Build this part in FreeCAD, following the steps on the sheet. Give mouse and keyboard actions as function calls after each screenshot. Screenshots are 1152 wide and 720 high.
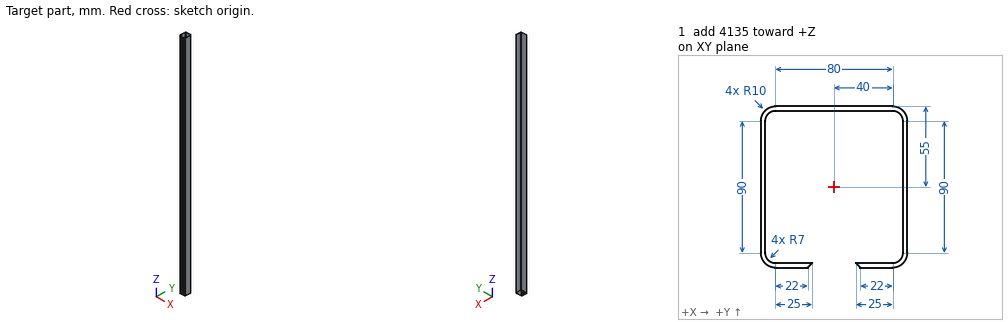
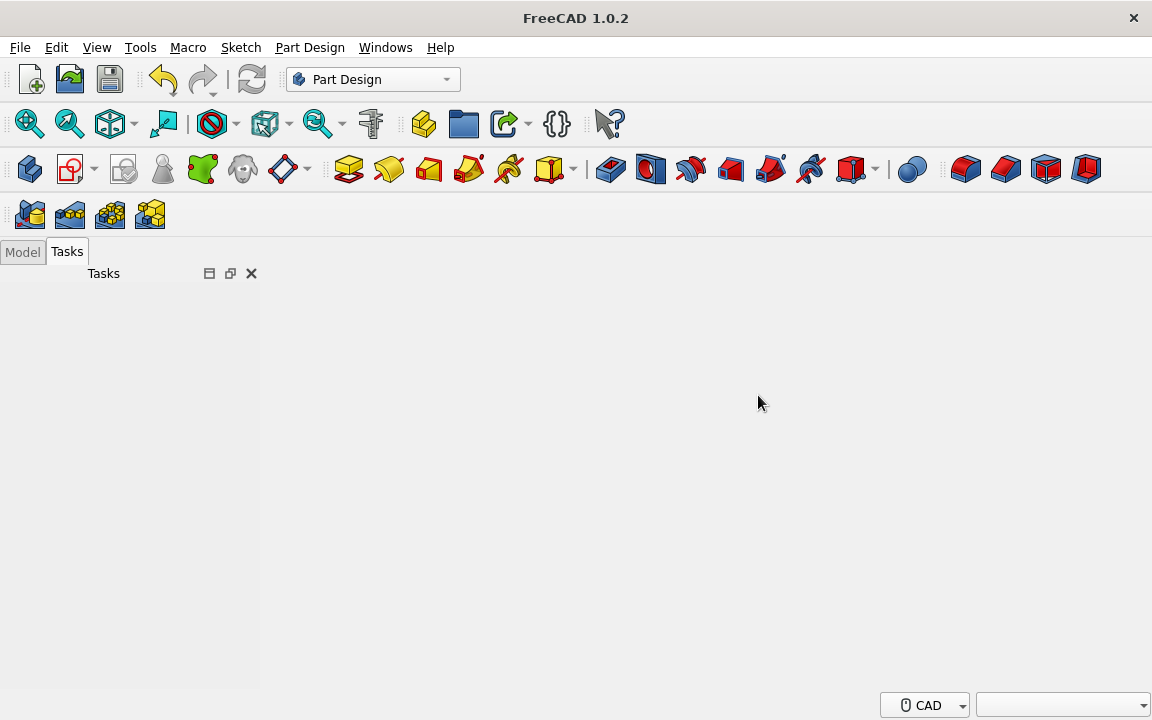
click(30, 80)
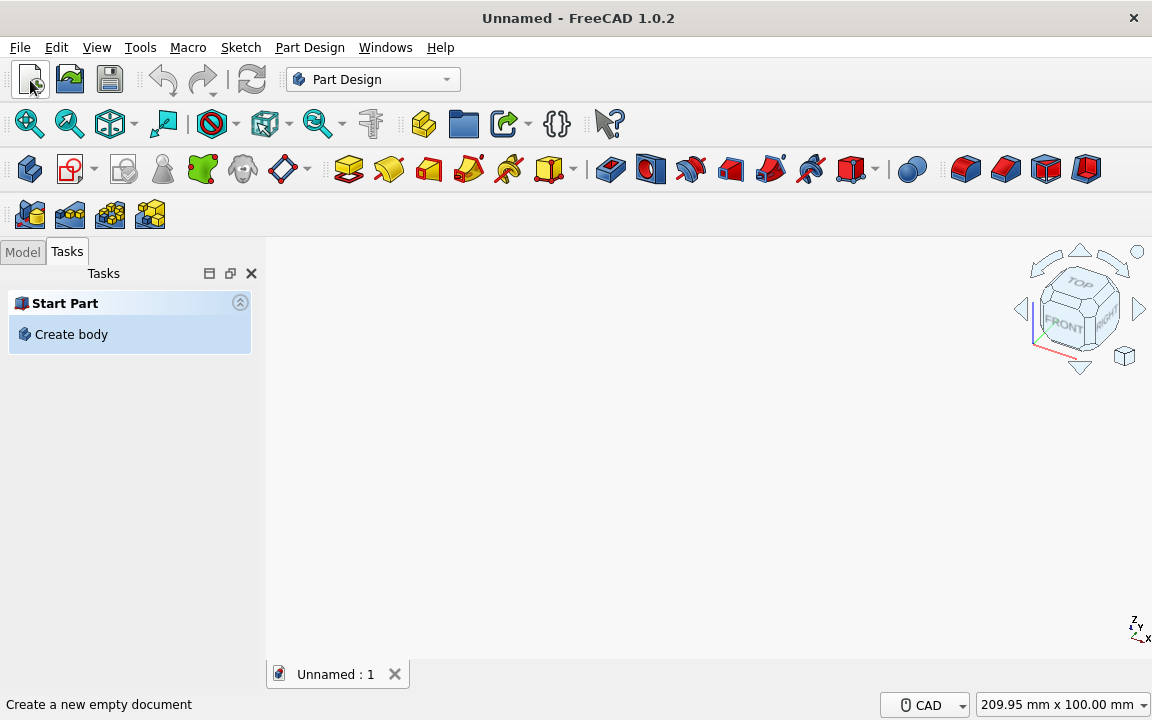
click(70, 170)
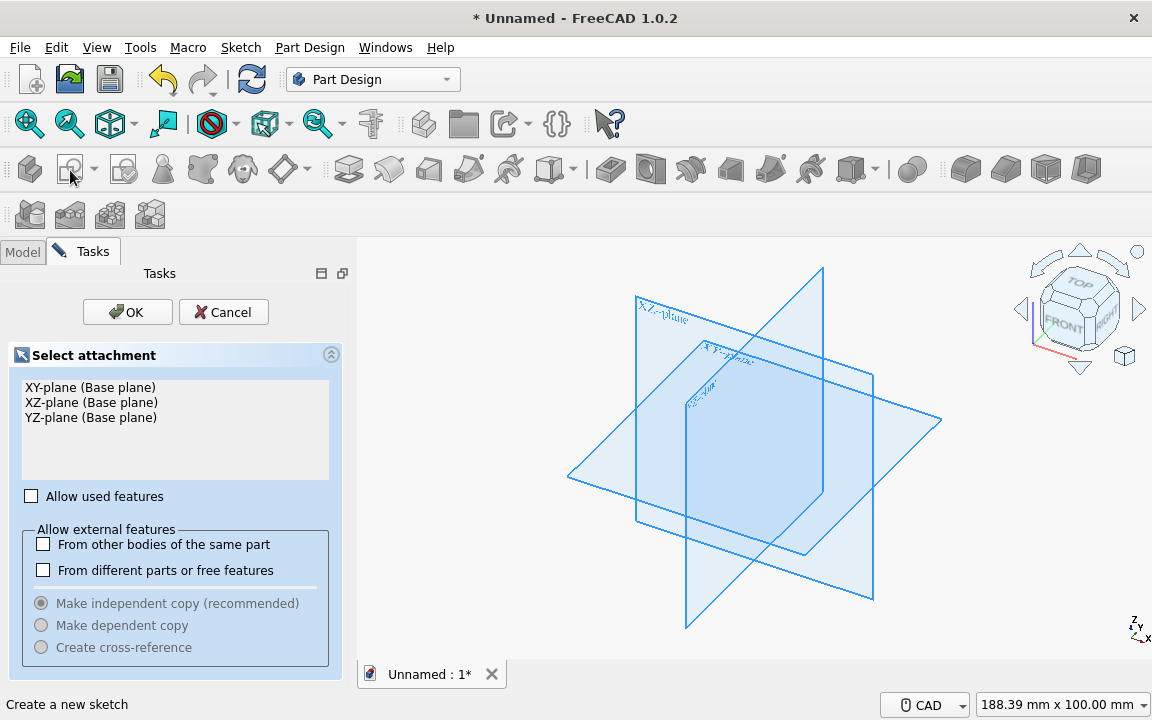
click(82, 388)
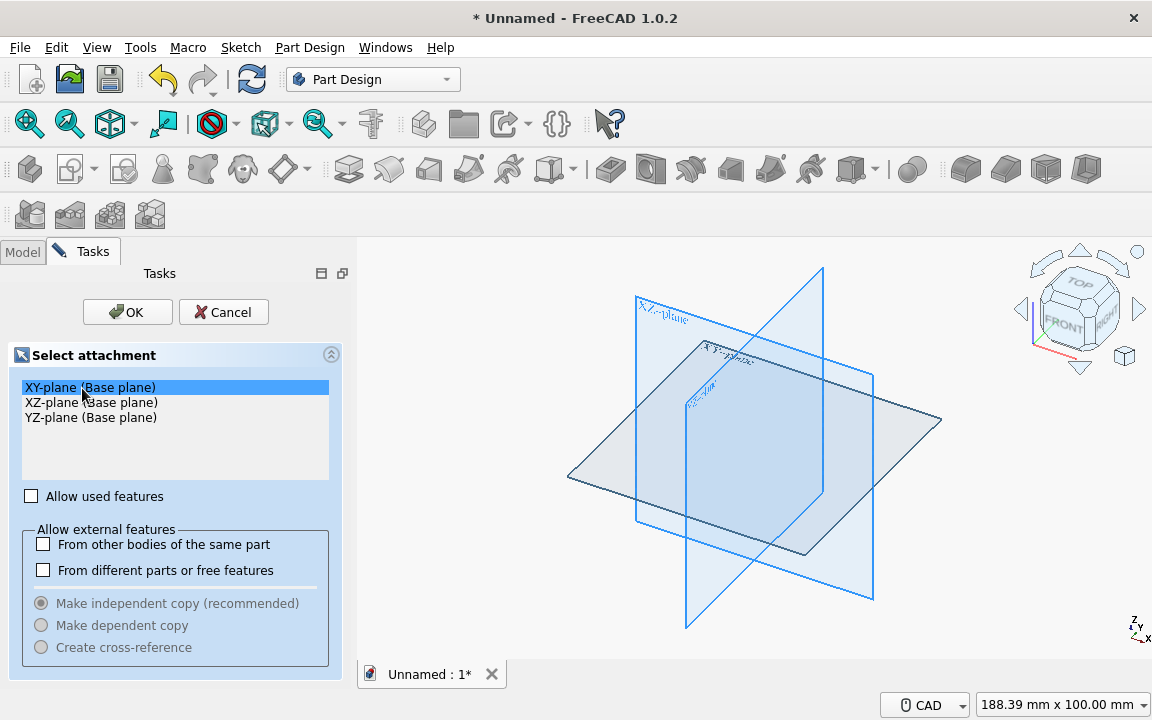
click(128, 312)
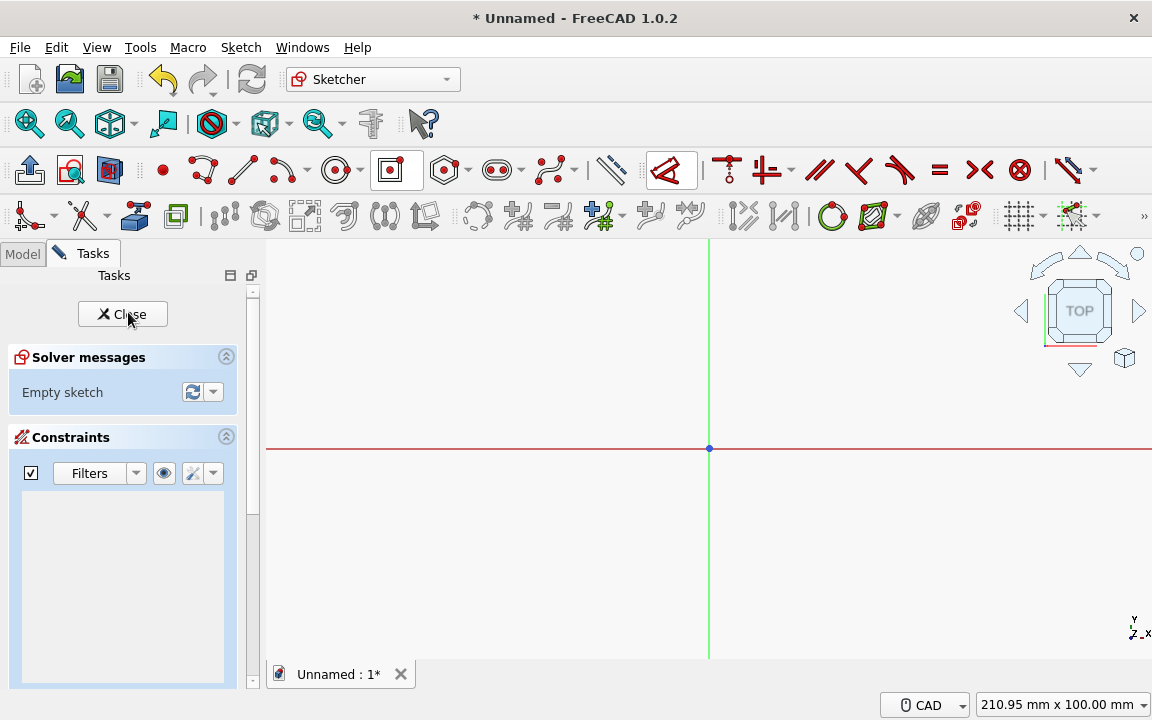
scroll(557, 449, down, 3)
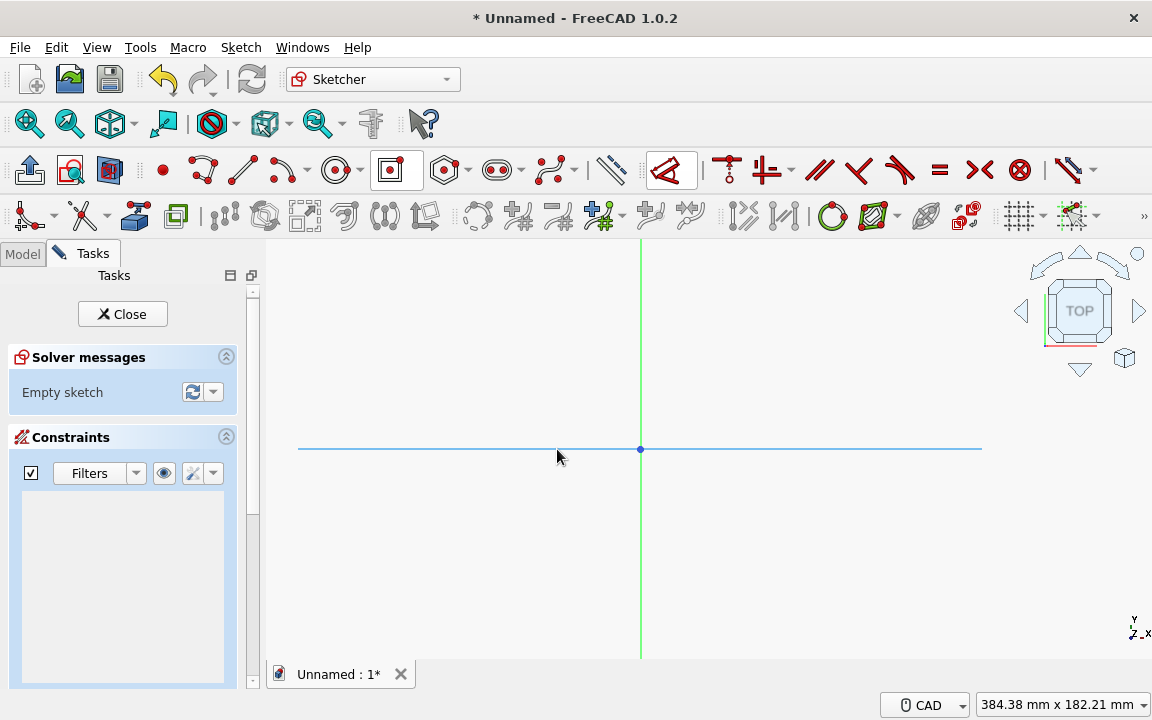
click(244, 170)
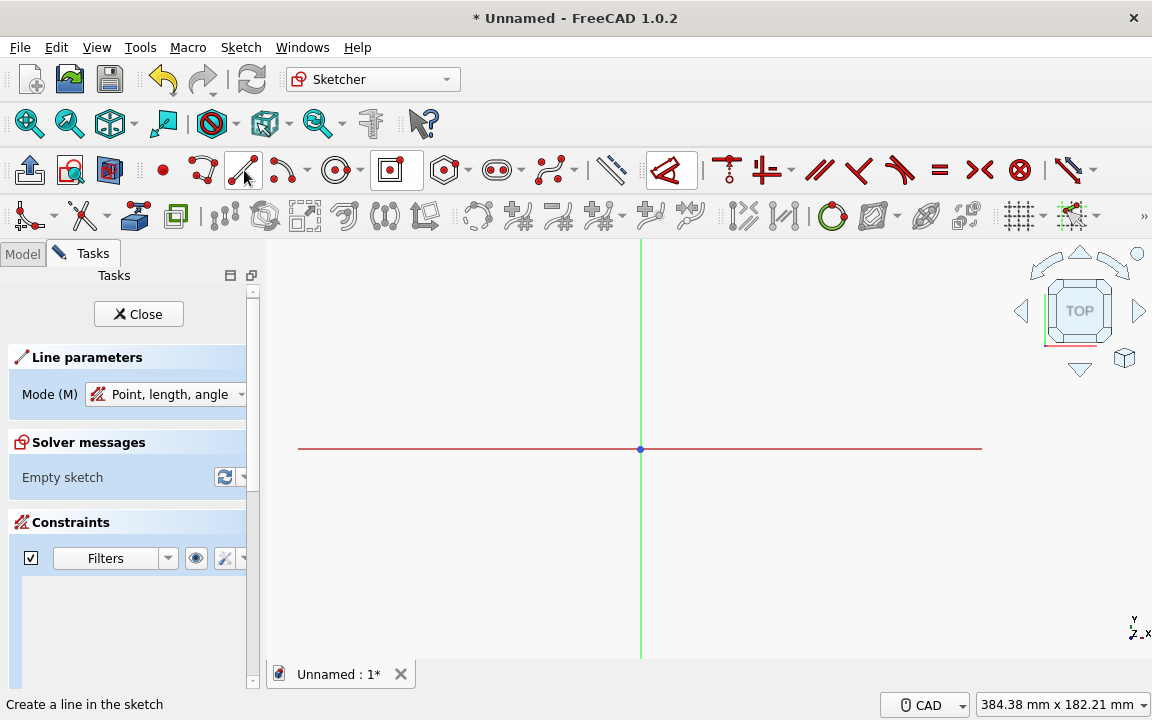
click(733, 322)
click(548, 322)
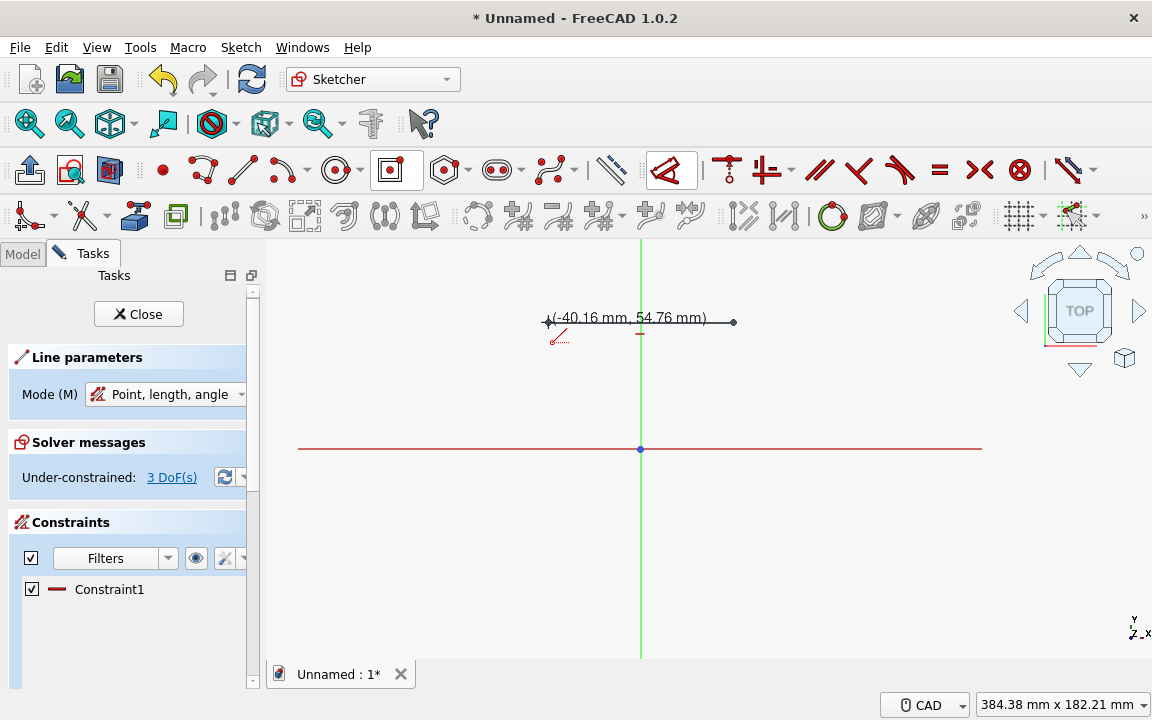
click(525, 346)
click(525, 553)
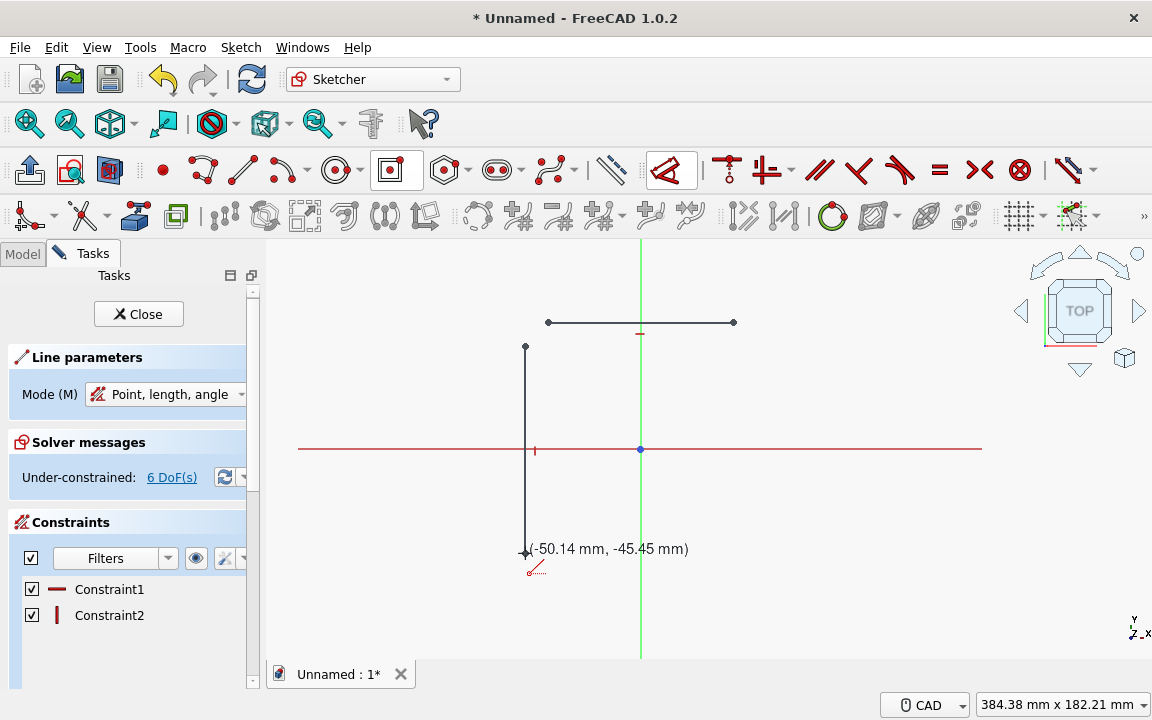
click(204, 170)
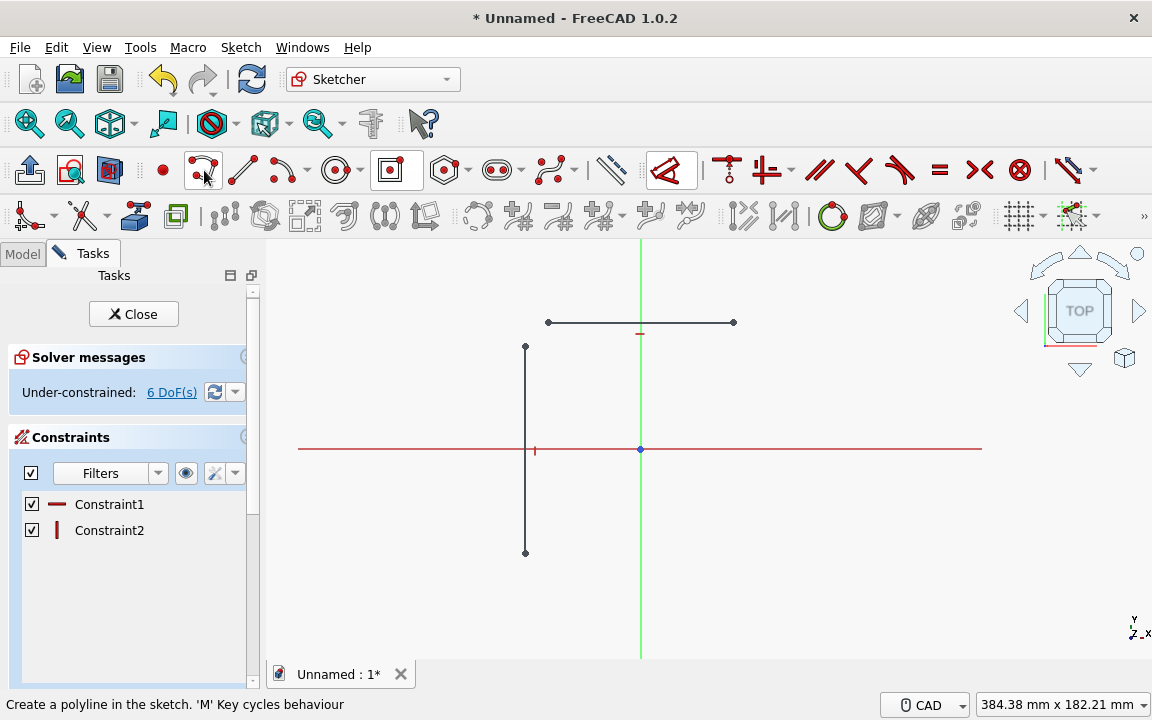
click(548, 576)
click(599, 576)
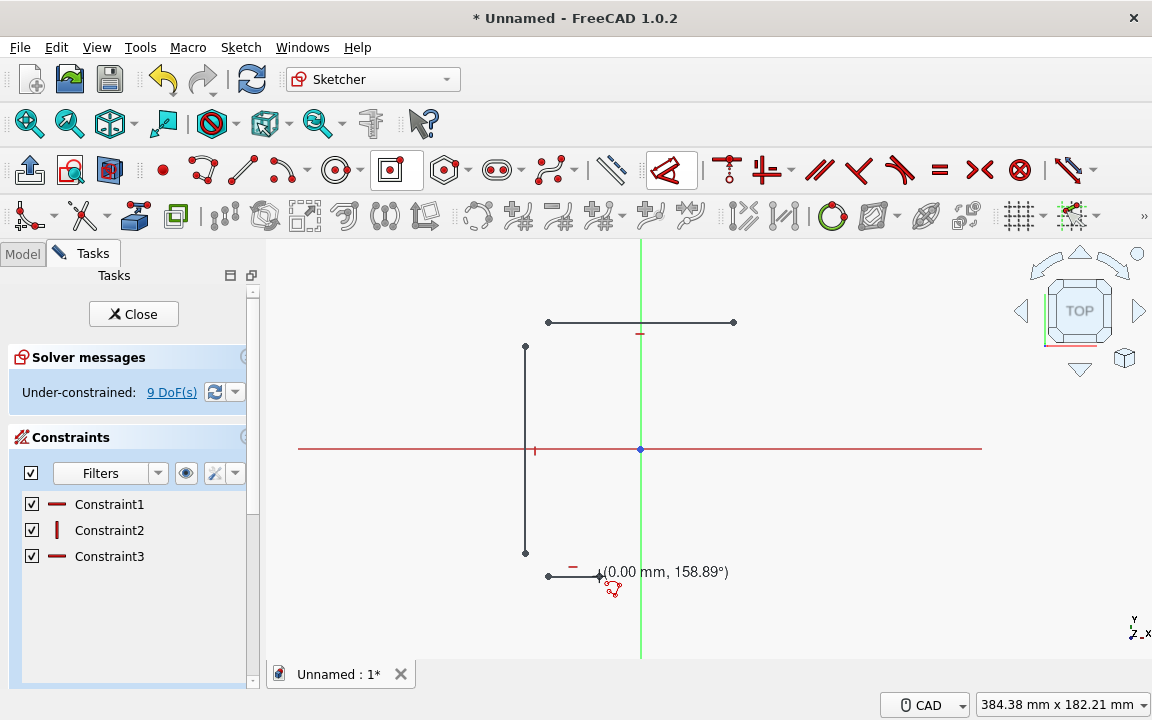
scroll(606, 569, up, 3)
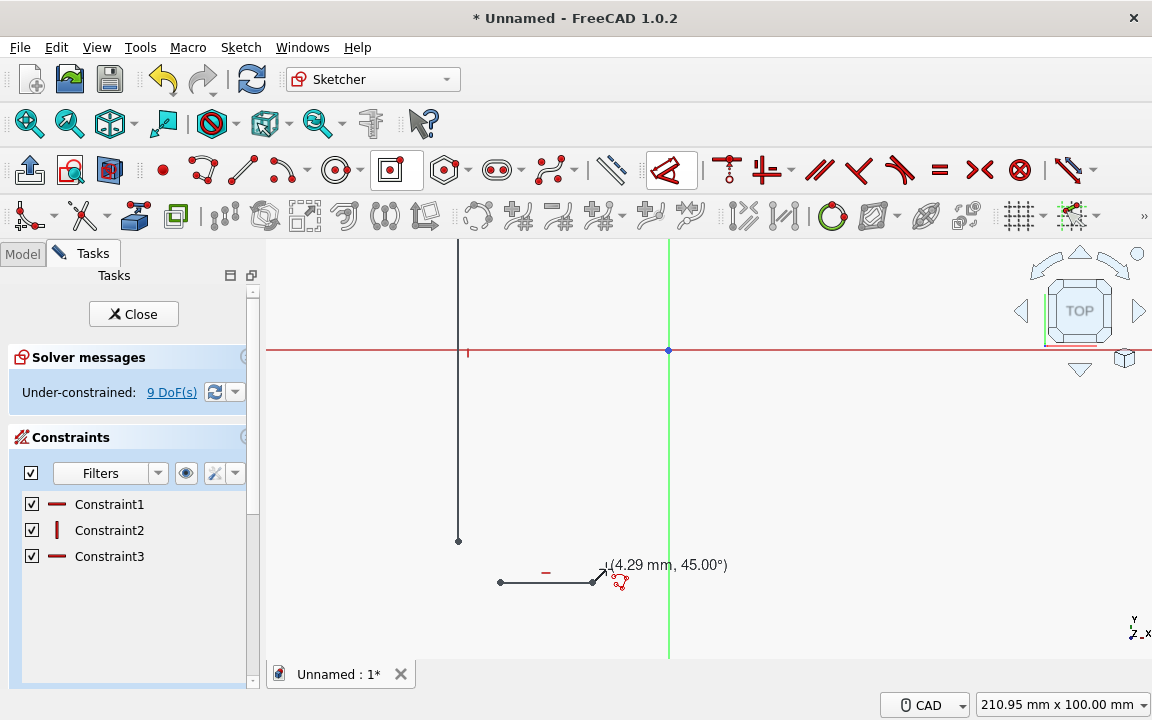
click(606, 569)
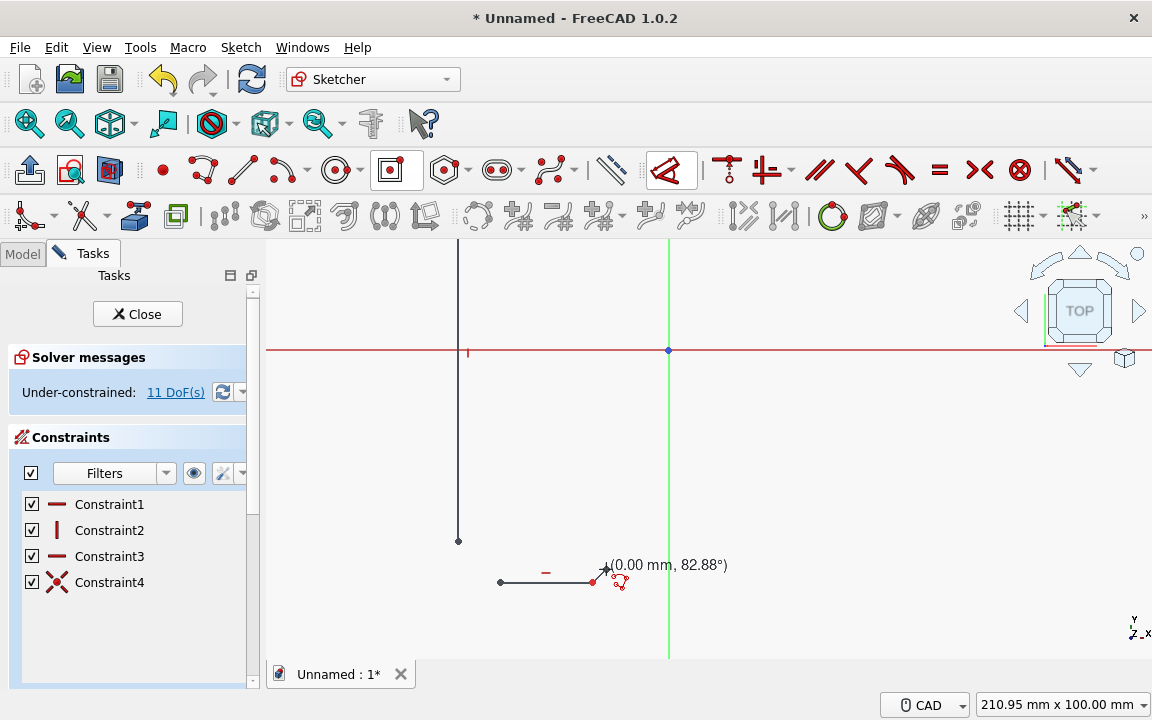
scroll(501, 569, up, 2)